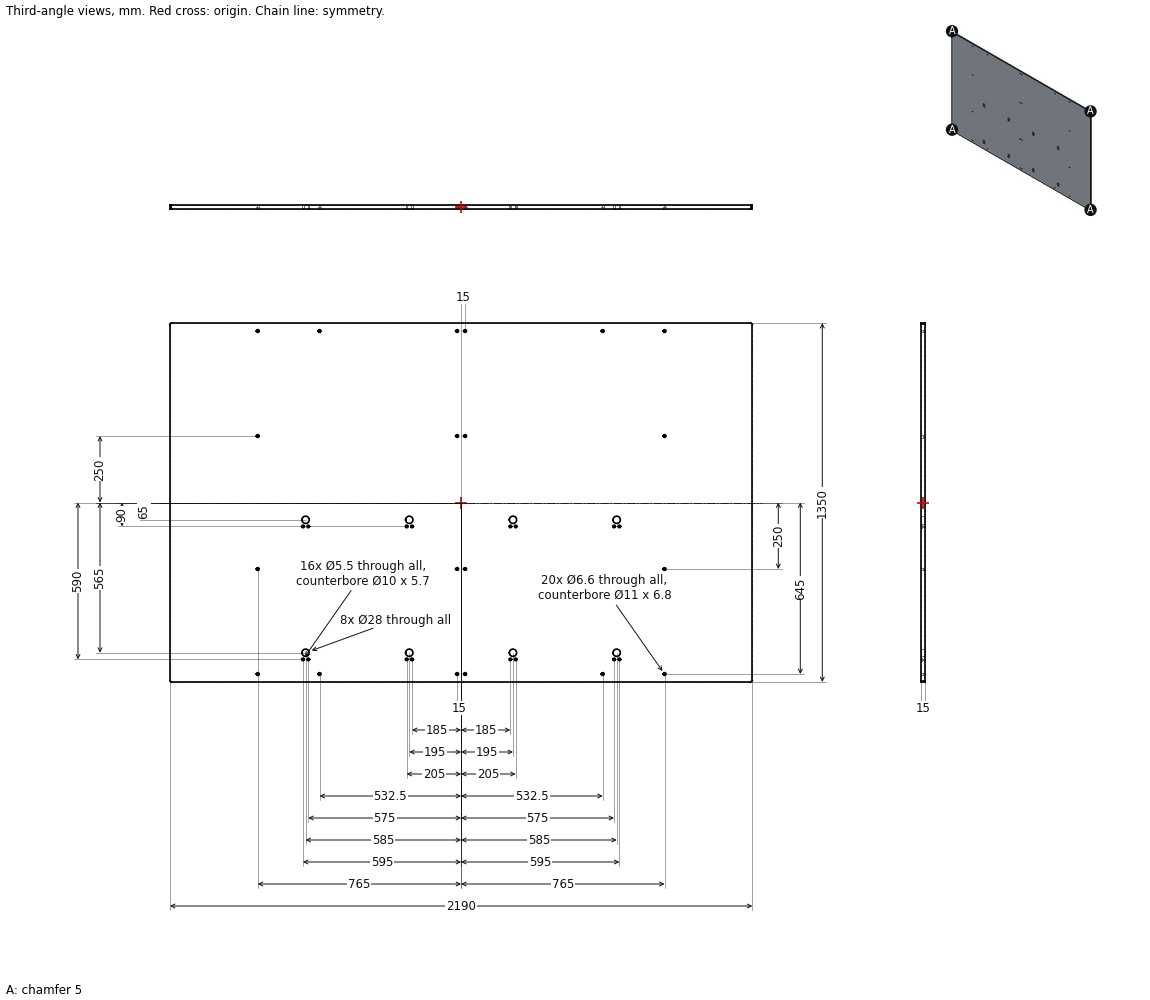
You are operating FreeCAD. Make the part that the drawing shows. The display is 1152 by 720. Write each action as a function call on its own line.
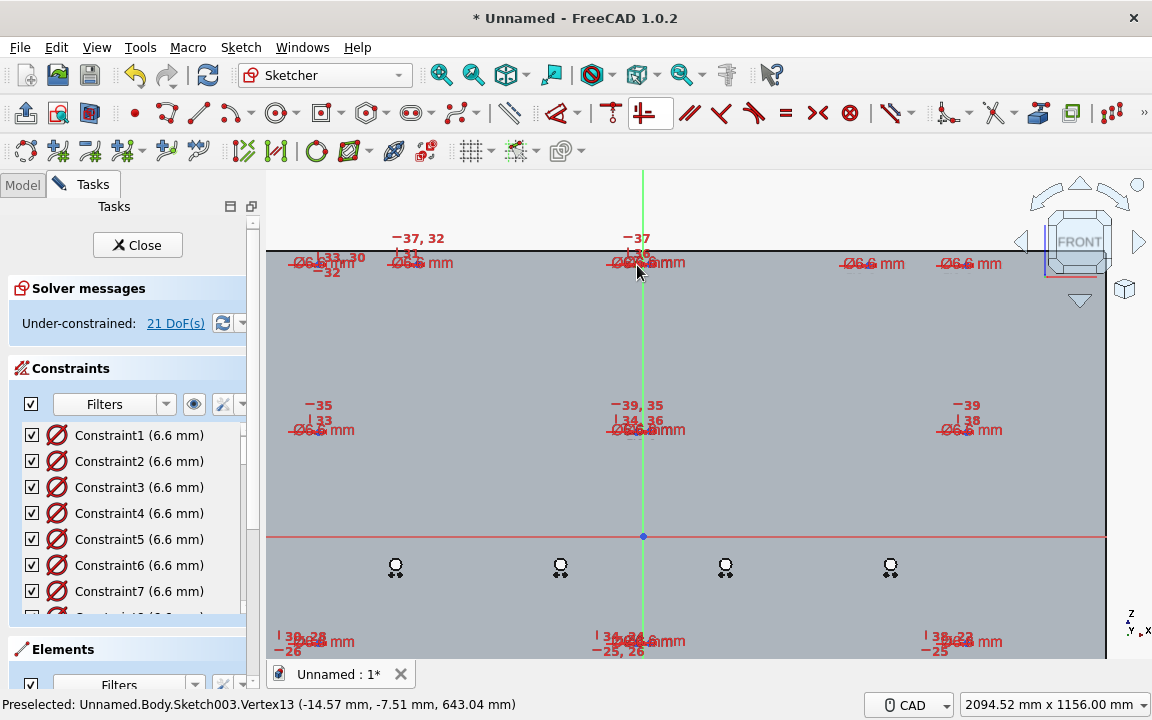
click(869, 266)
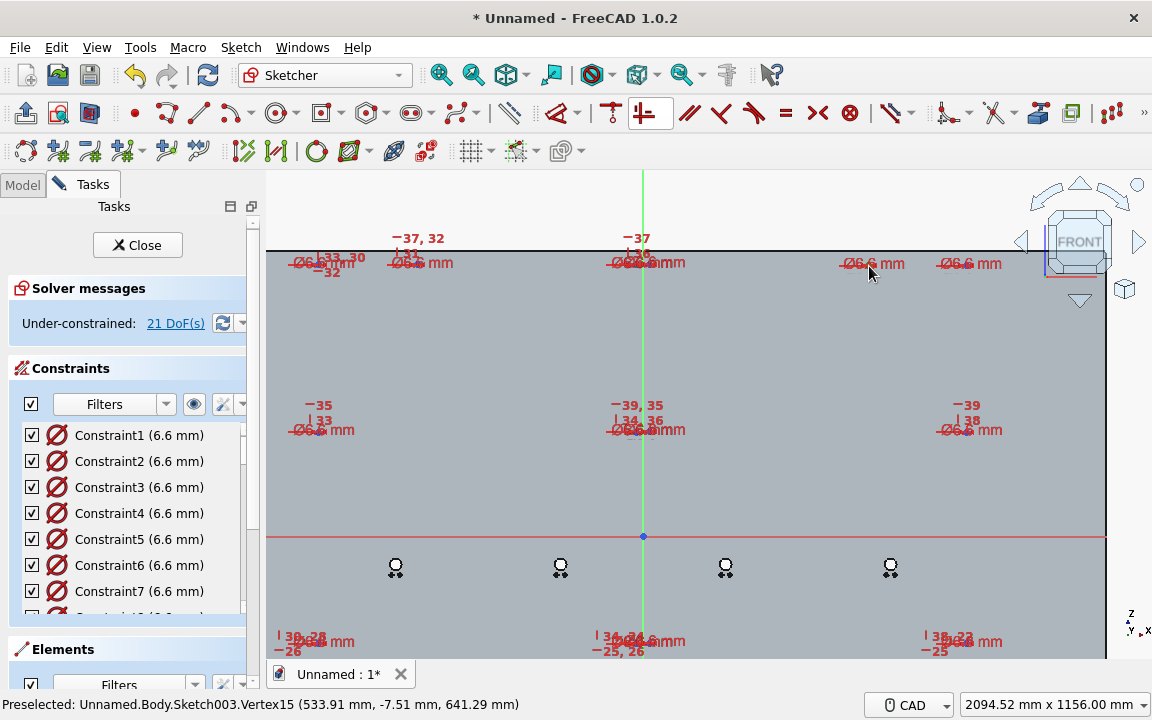
click(668, 114)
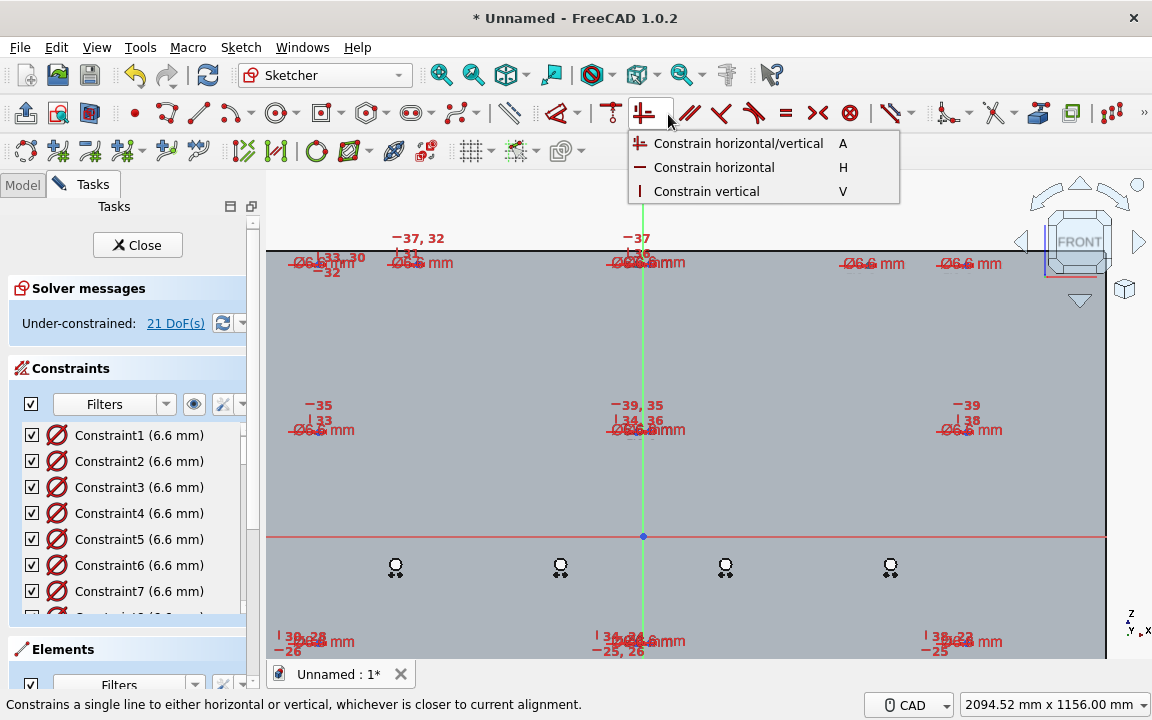
click(764, 167)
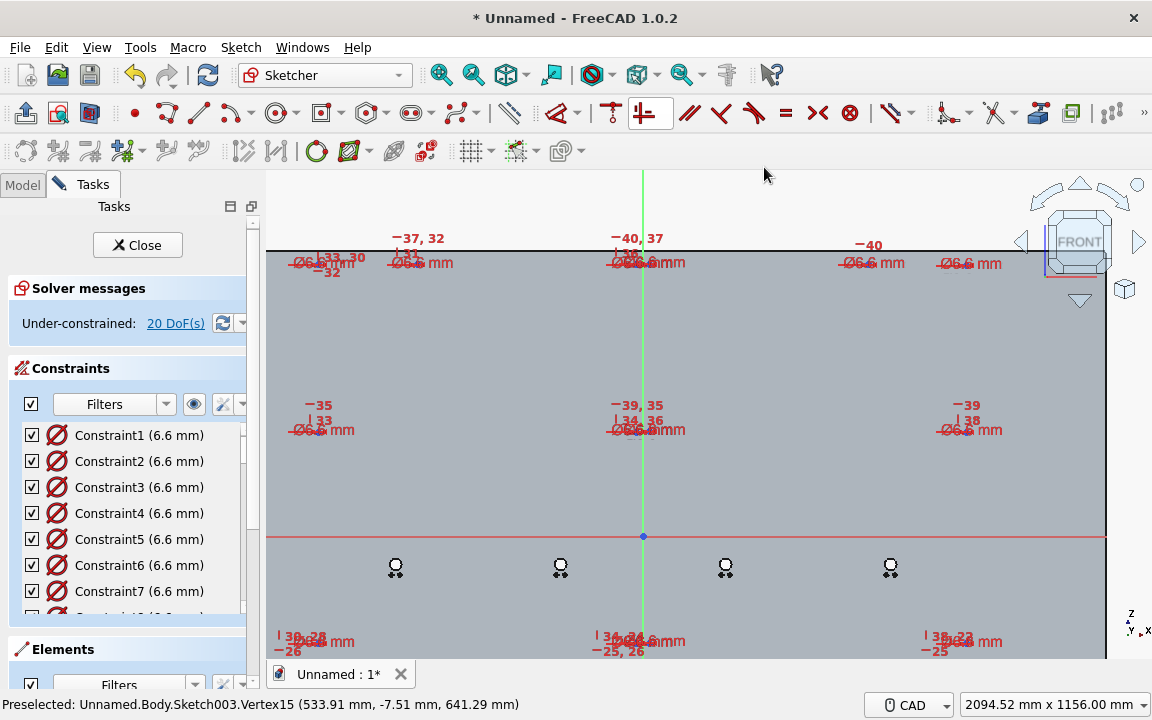
click(967, 432)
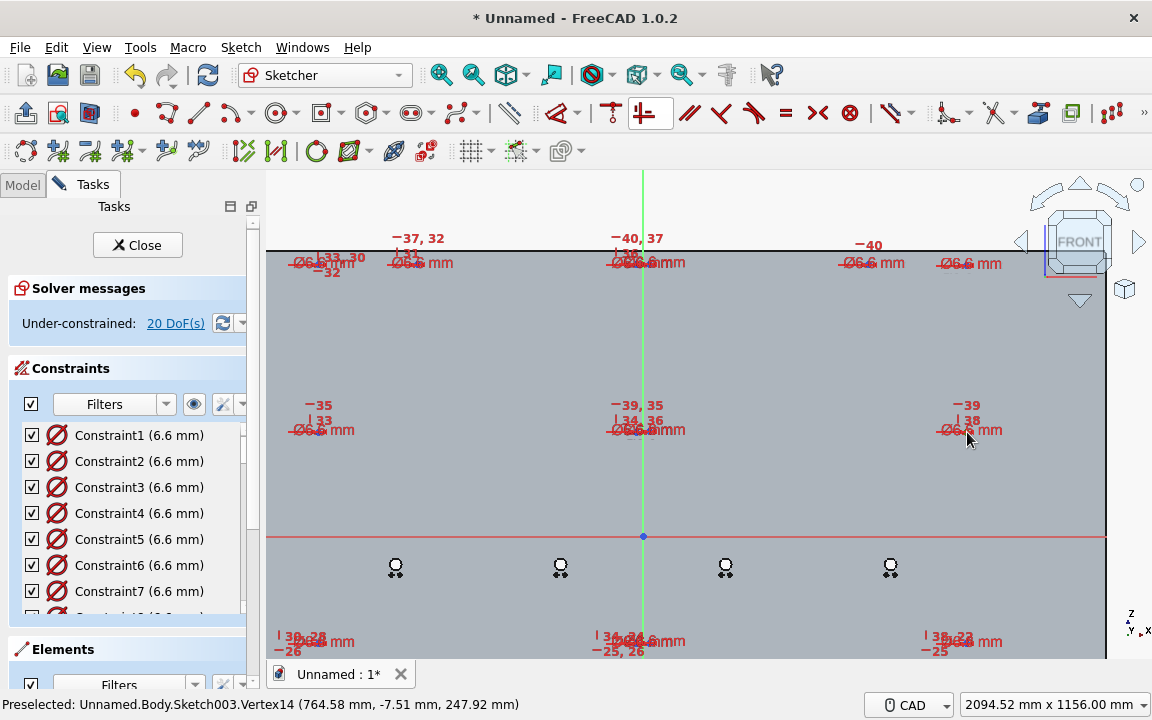
click(966, 266)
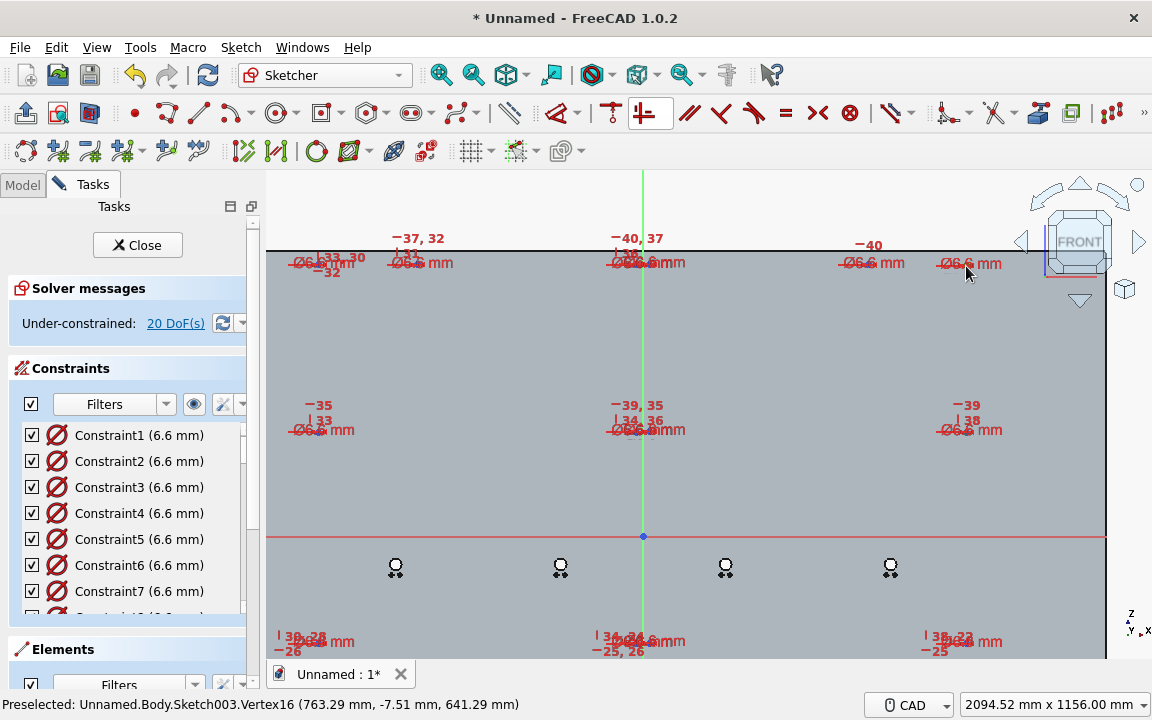
click(668, 114)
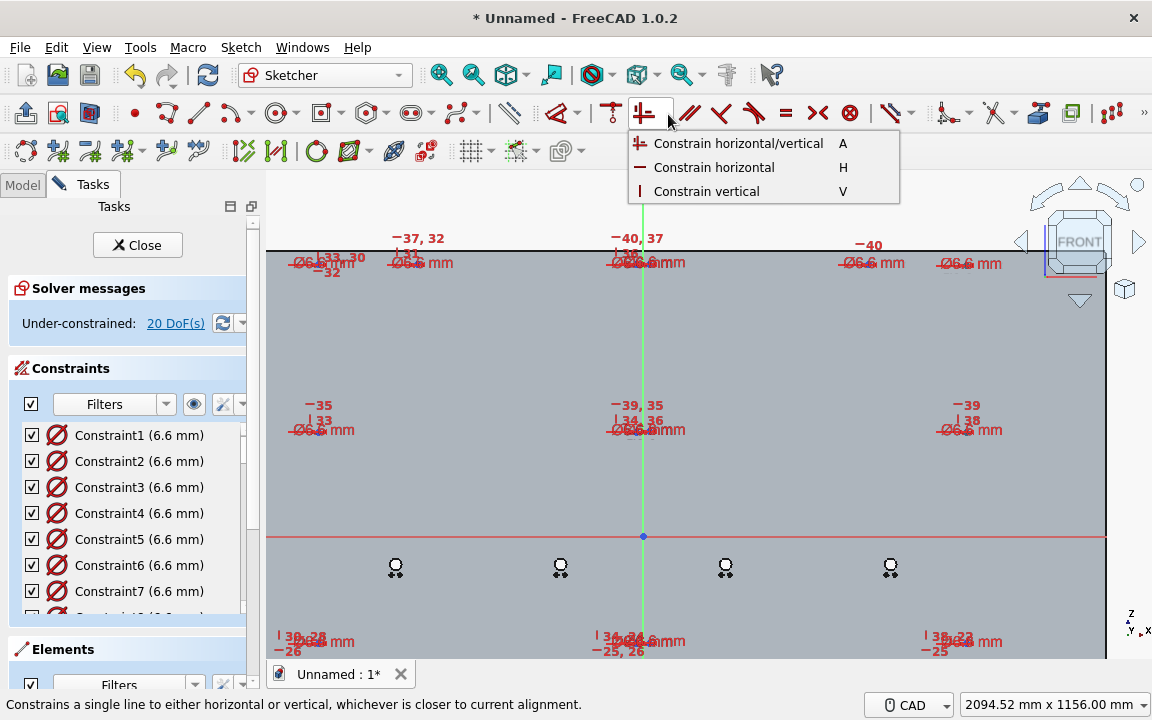
click(764, 191)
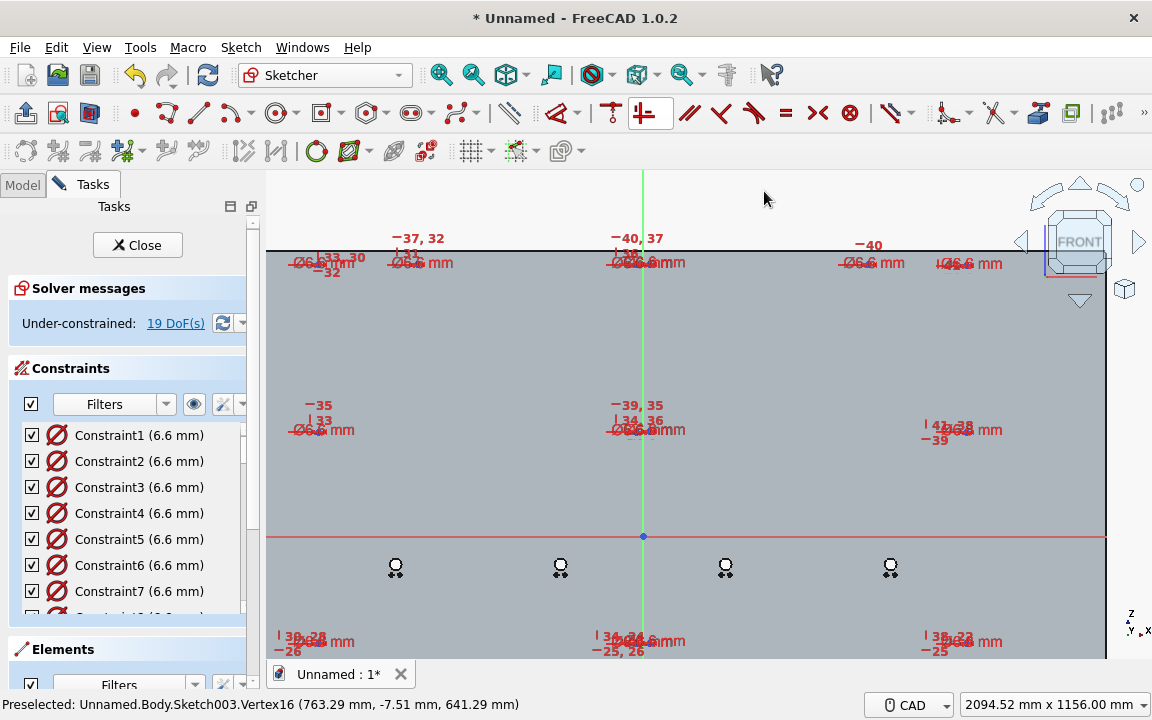
click(869, 265)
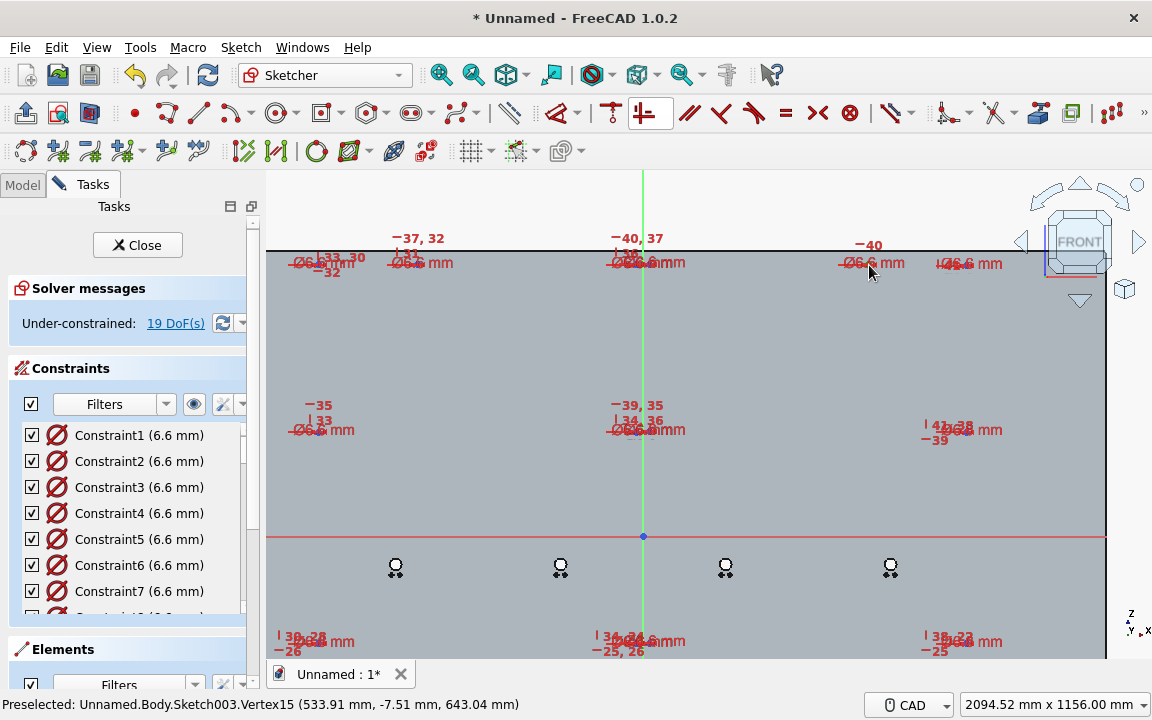
click(967, 266)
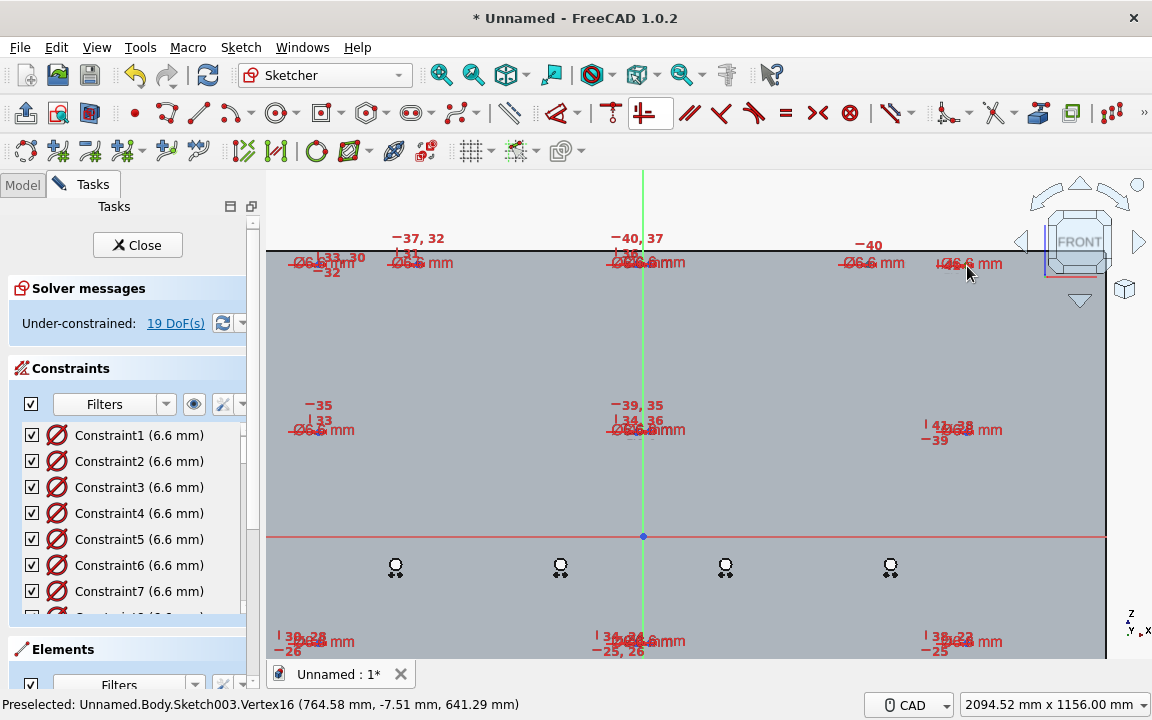
key(h)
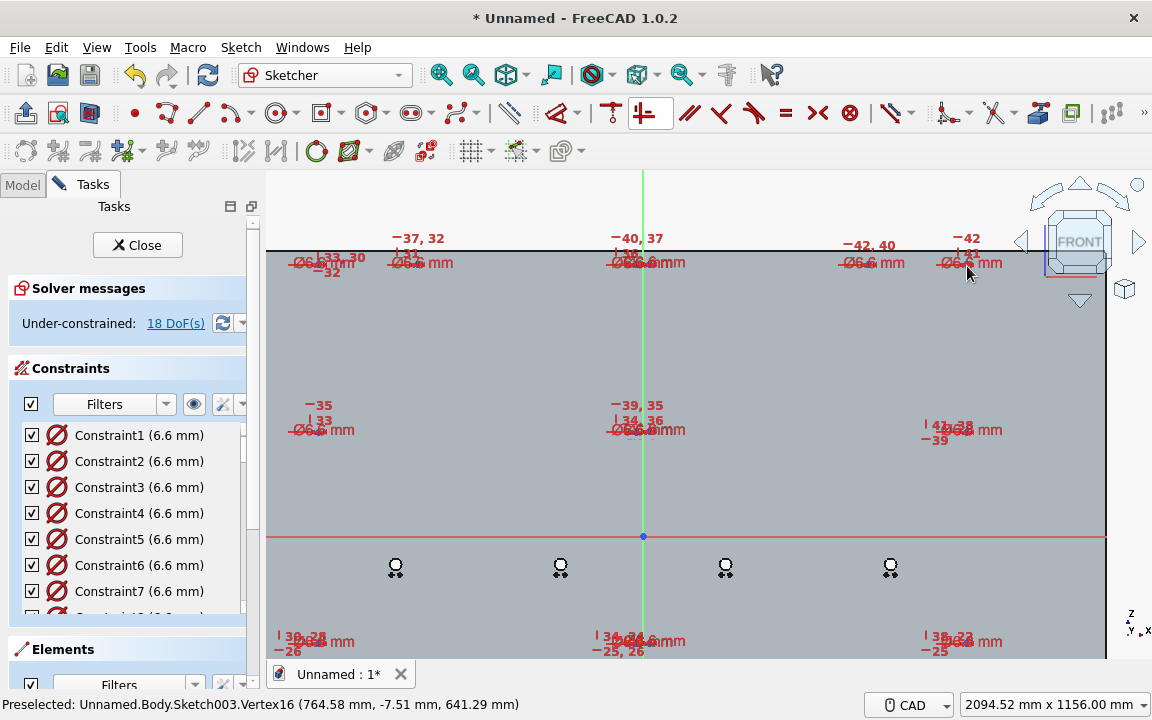
click(637, 265)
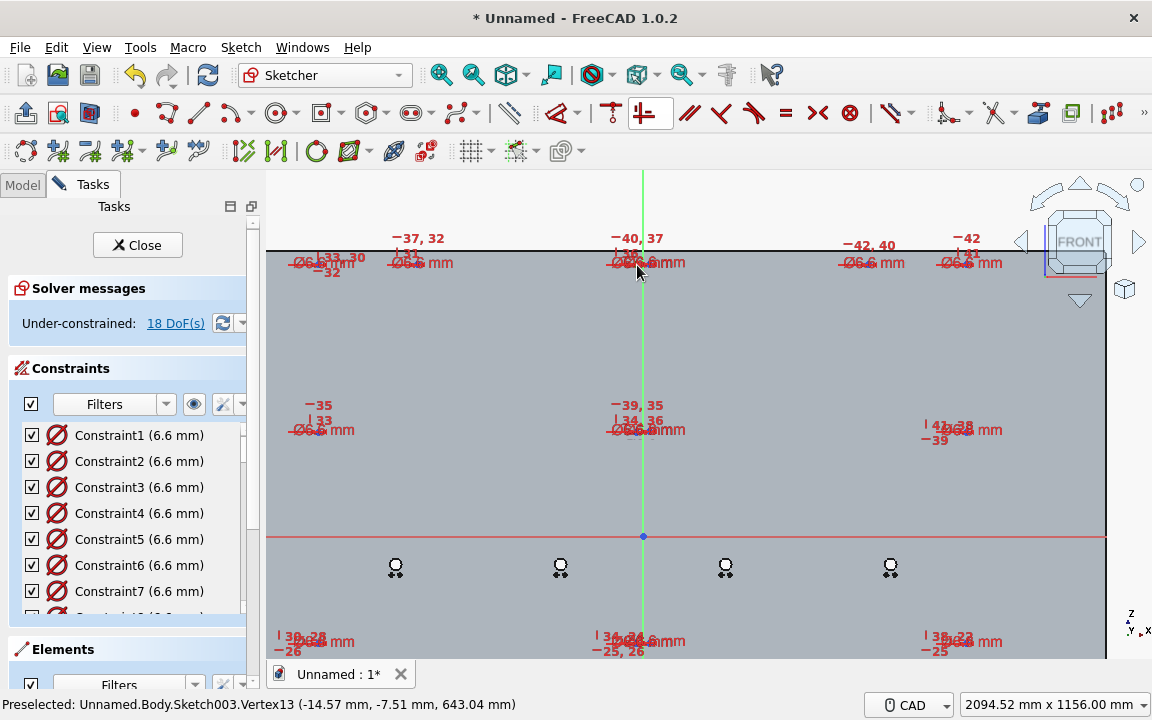
click(649, 264)